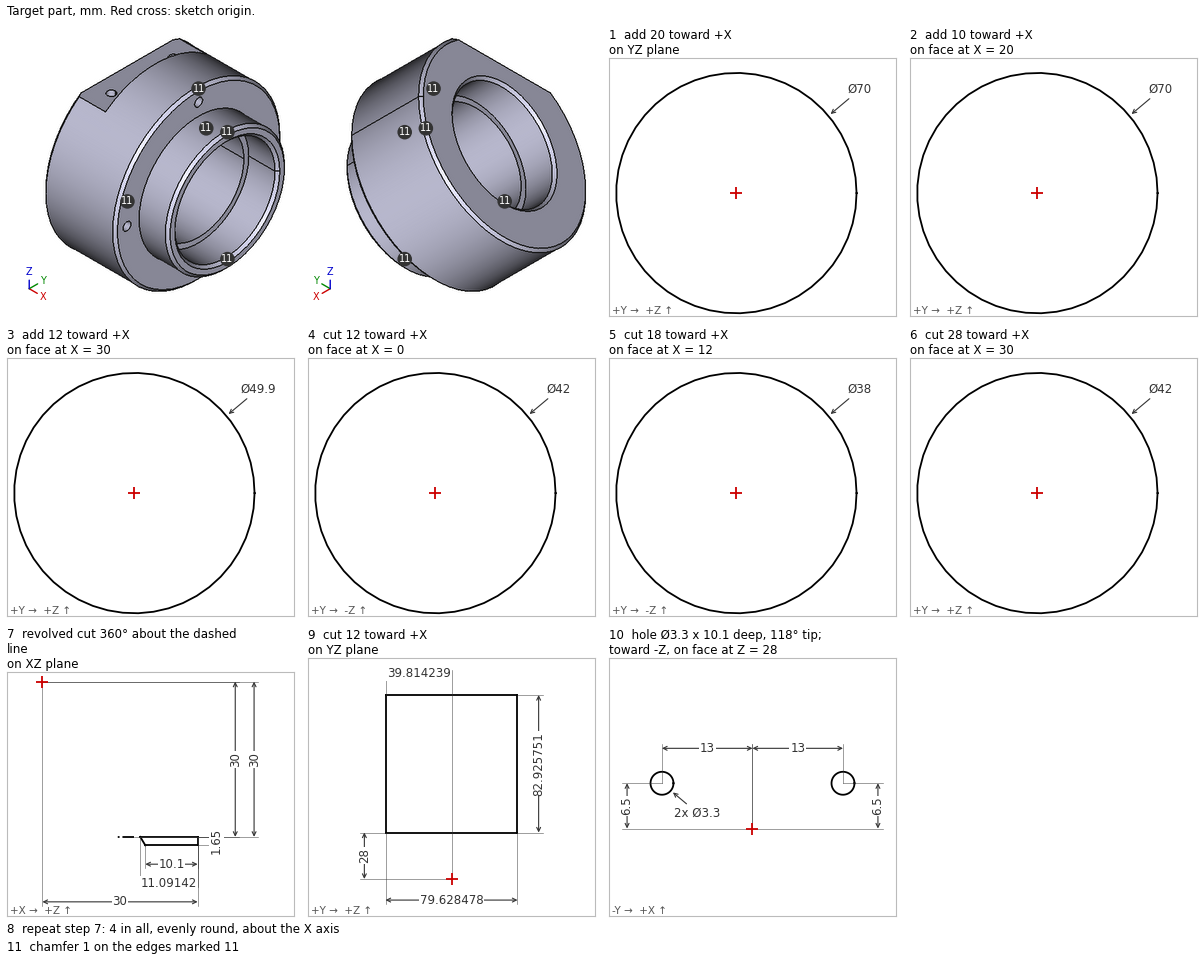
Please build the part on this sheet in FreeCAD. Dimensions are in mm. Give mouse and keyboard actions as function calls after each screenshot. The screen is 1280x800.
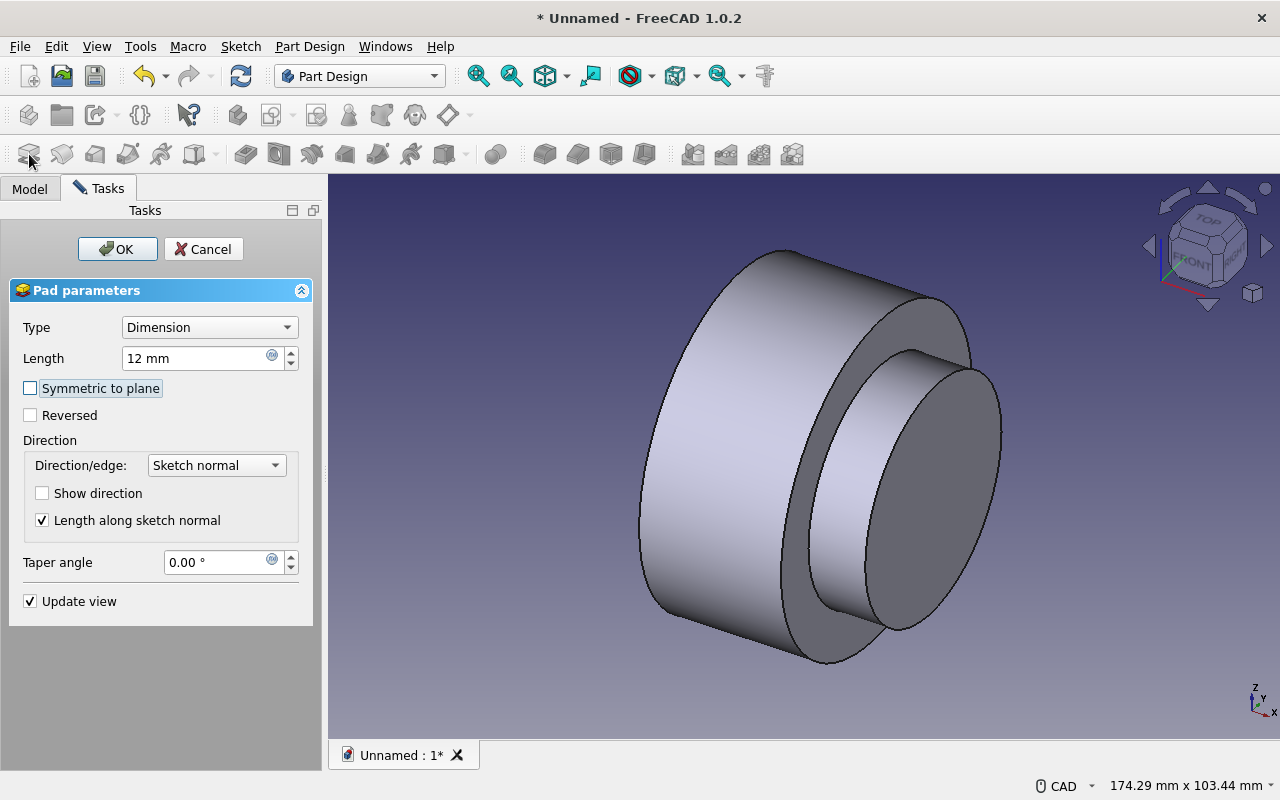
click(118, 249)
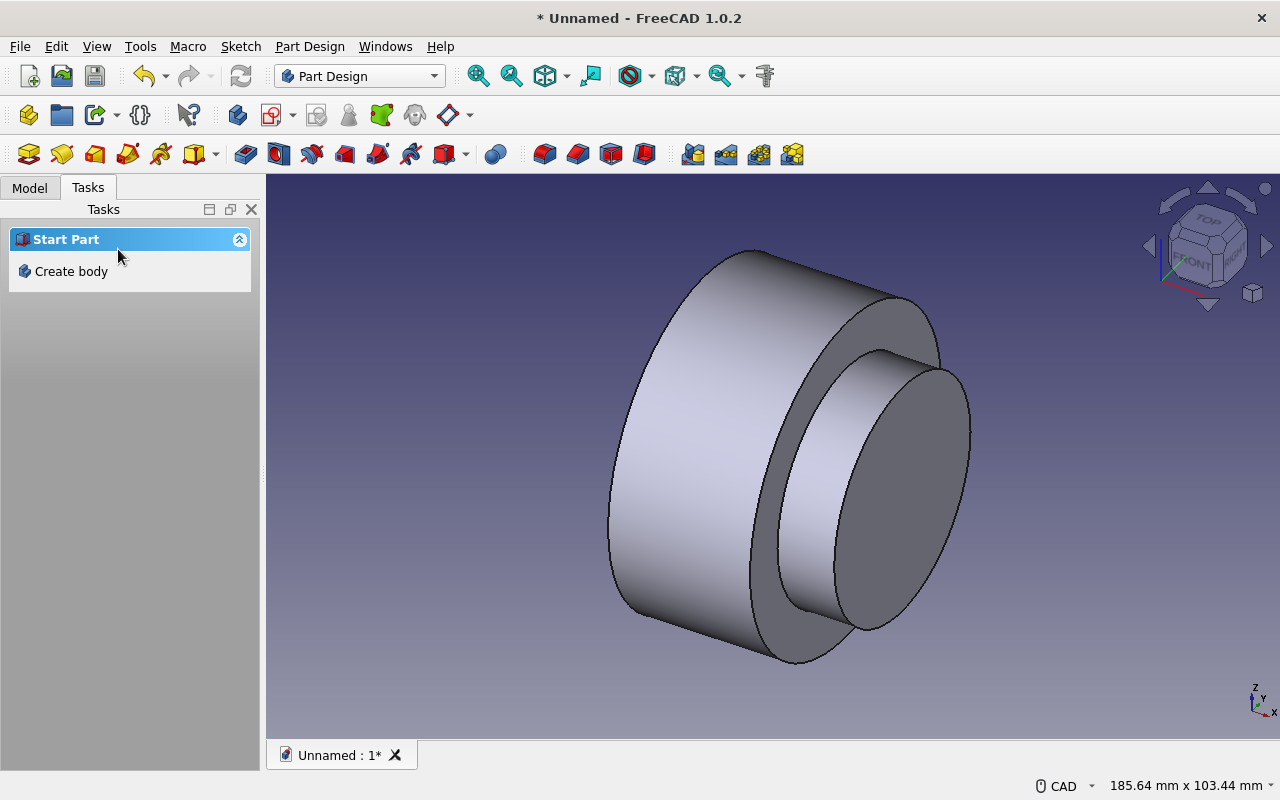
click(479, 76)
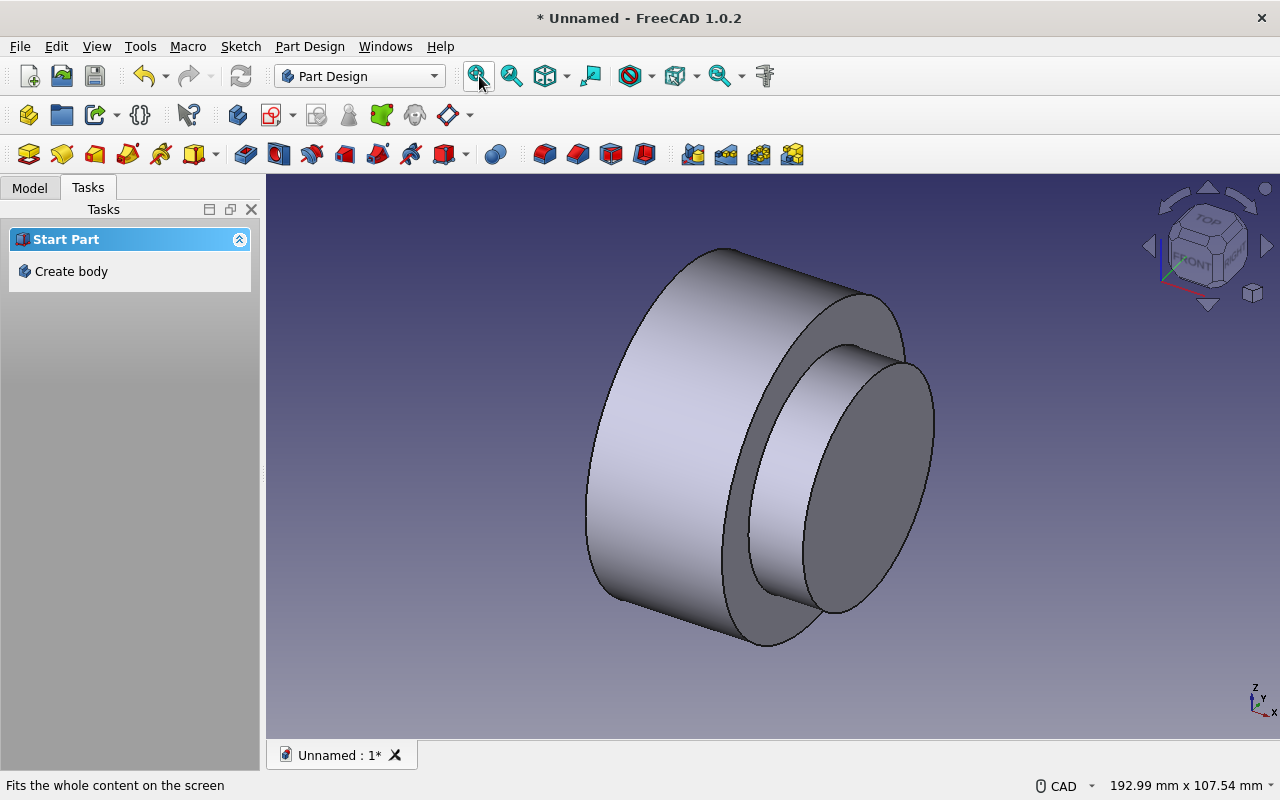
key(6)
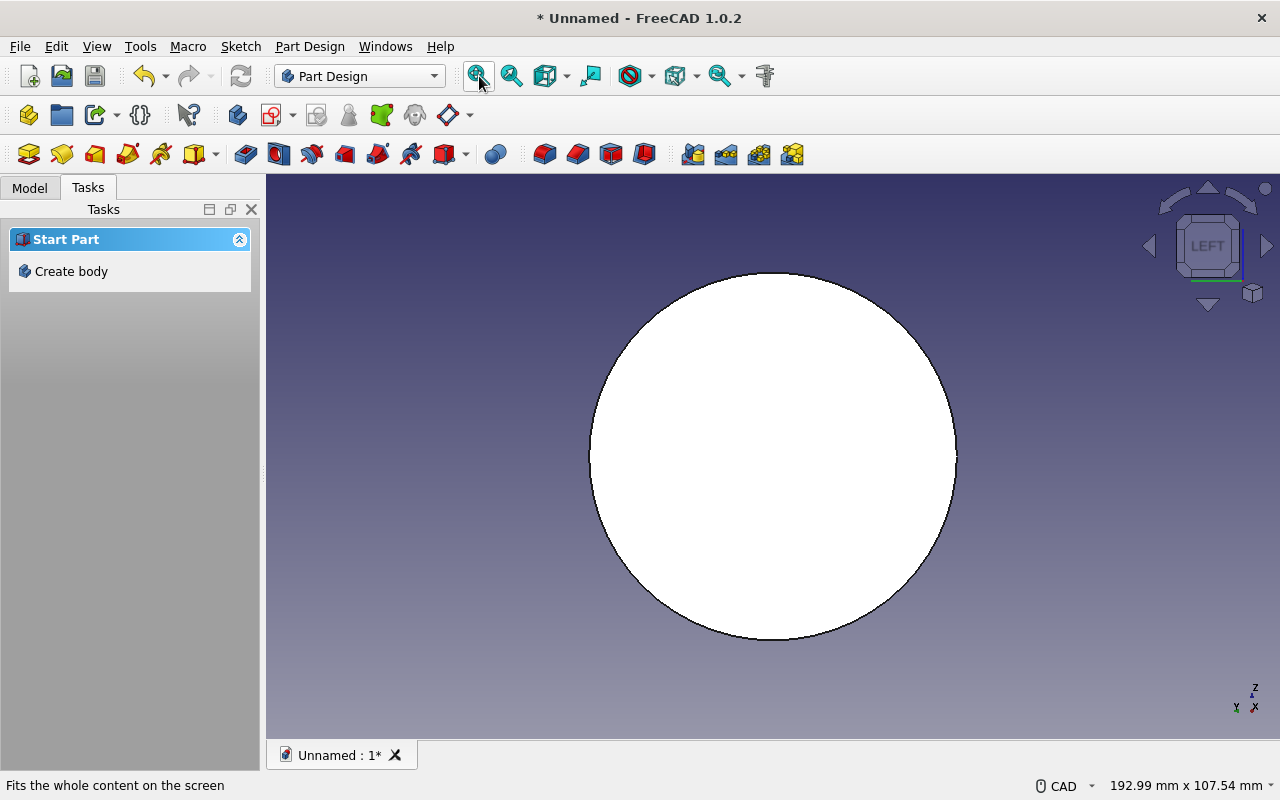
click(773, 455)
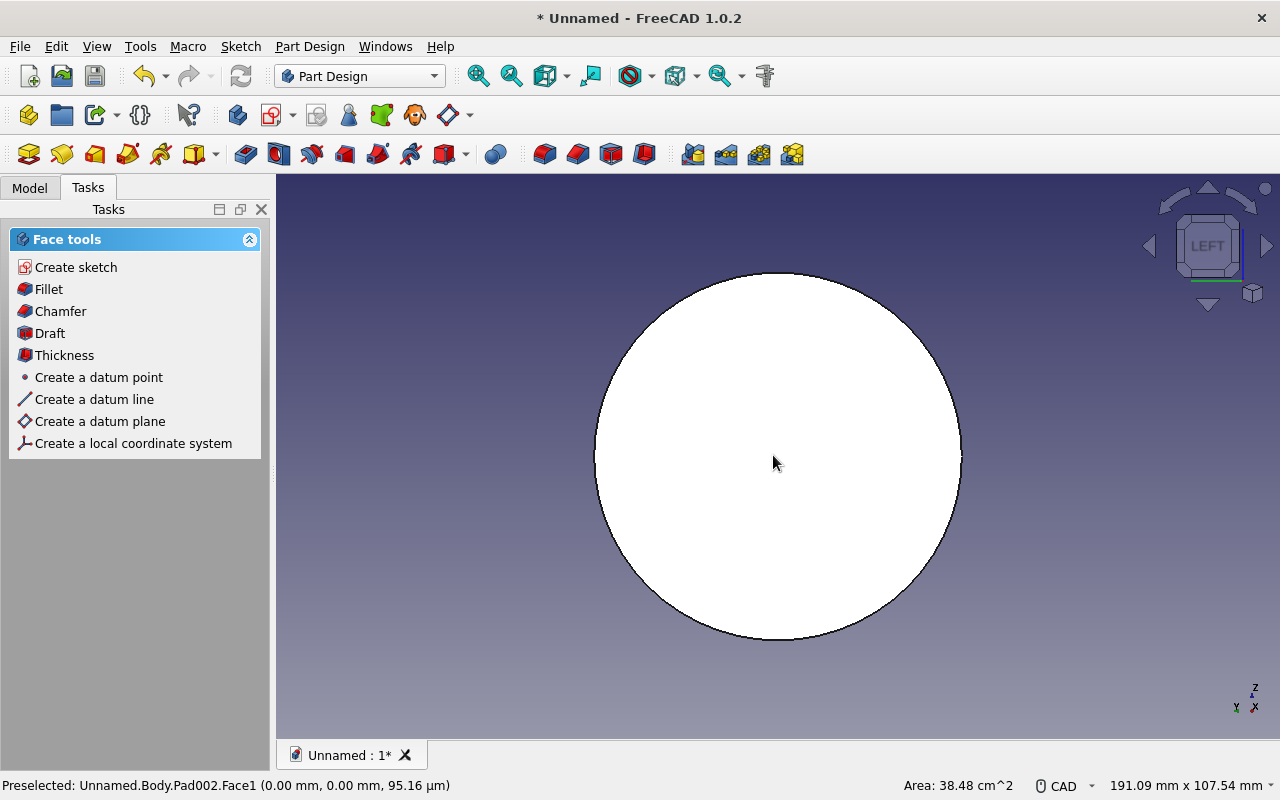
click(270, 116)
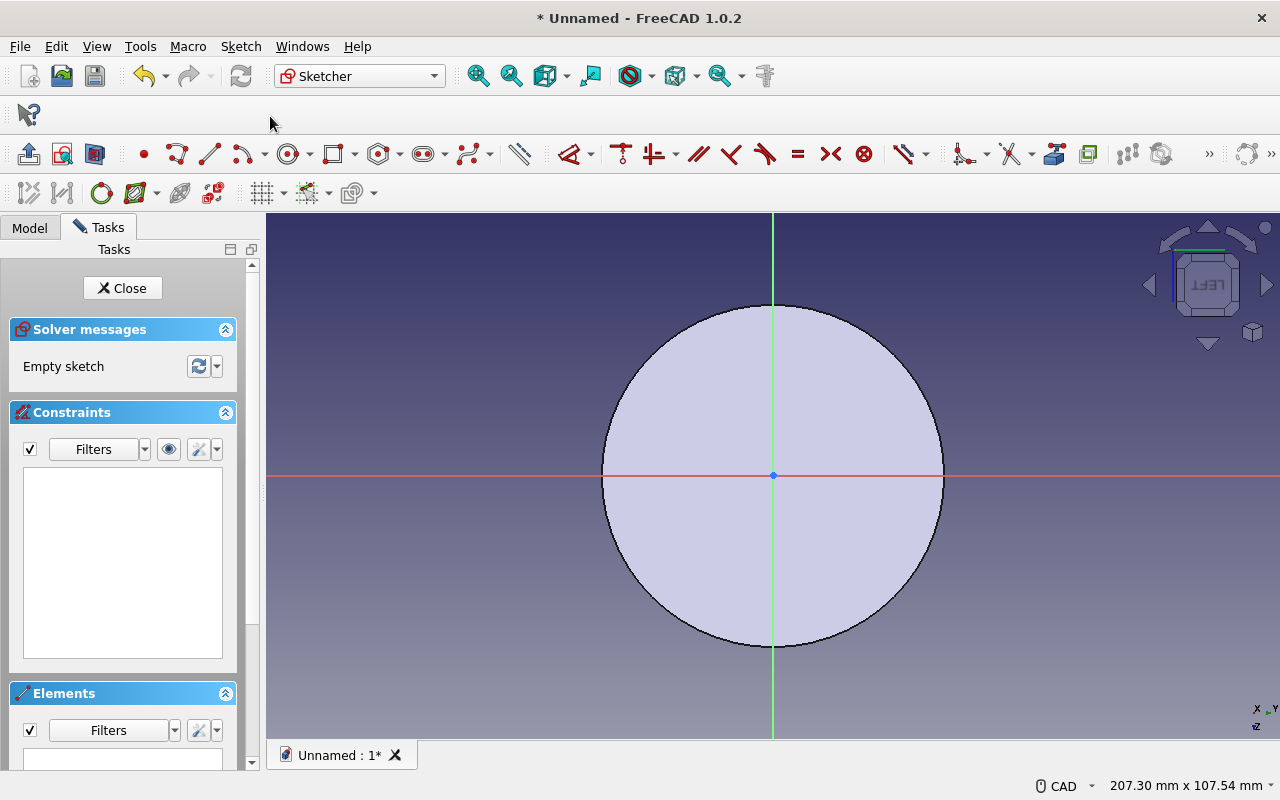
scroll(912, 476, up, 2)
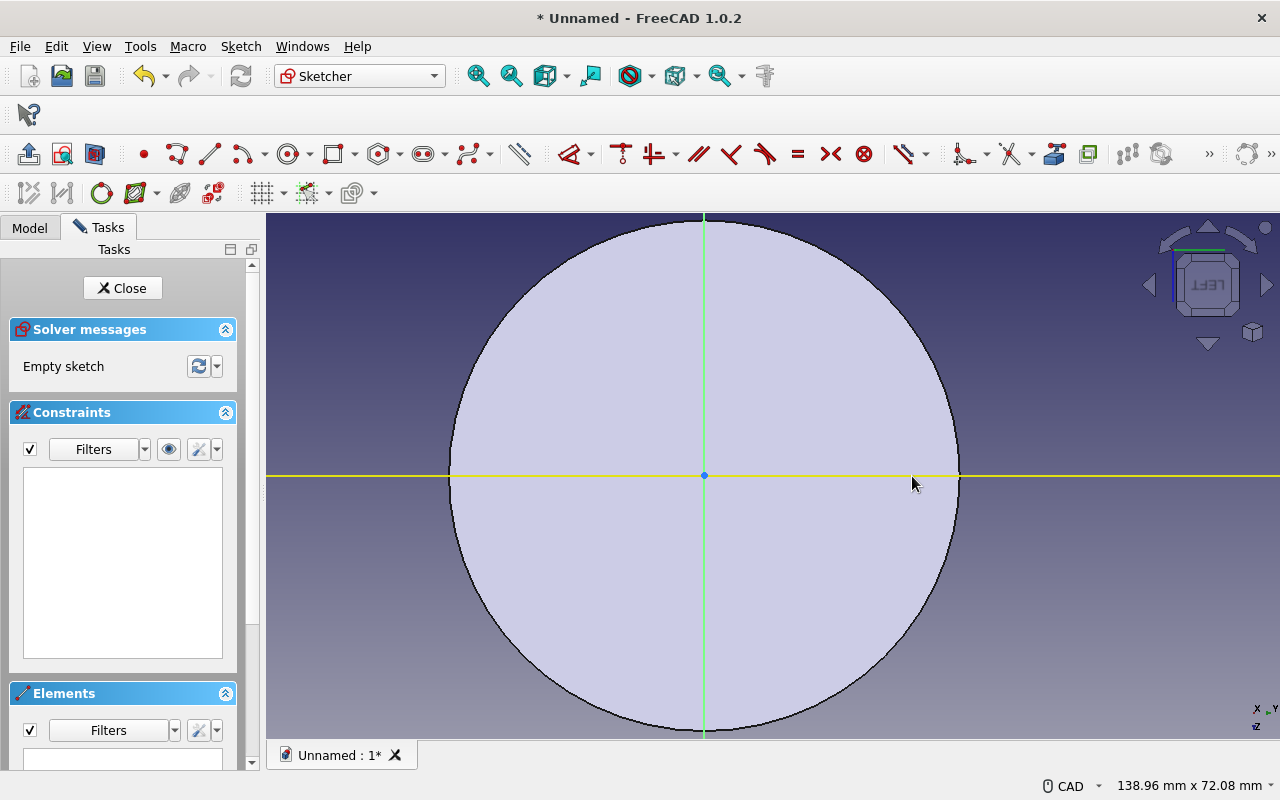
key(g)
key(c)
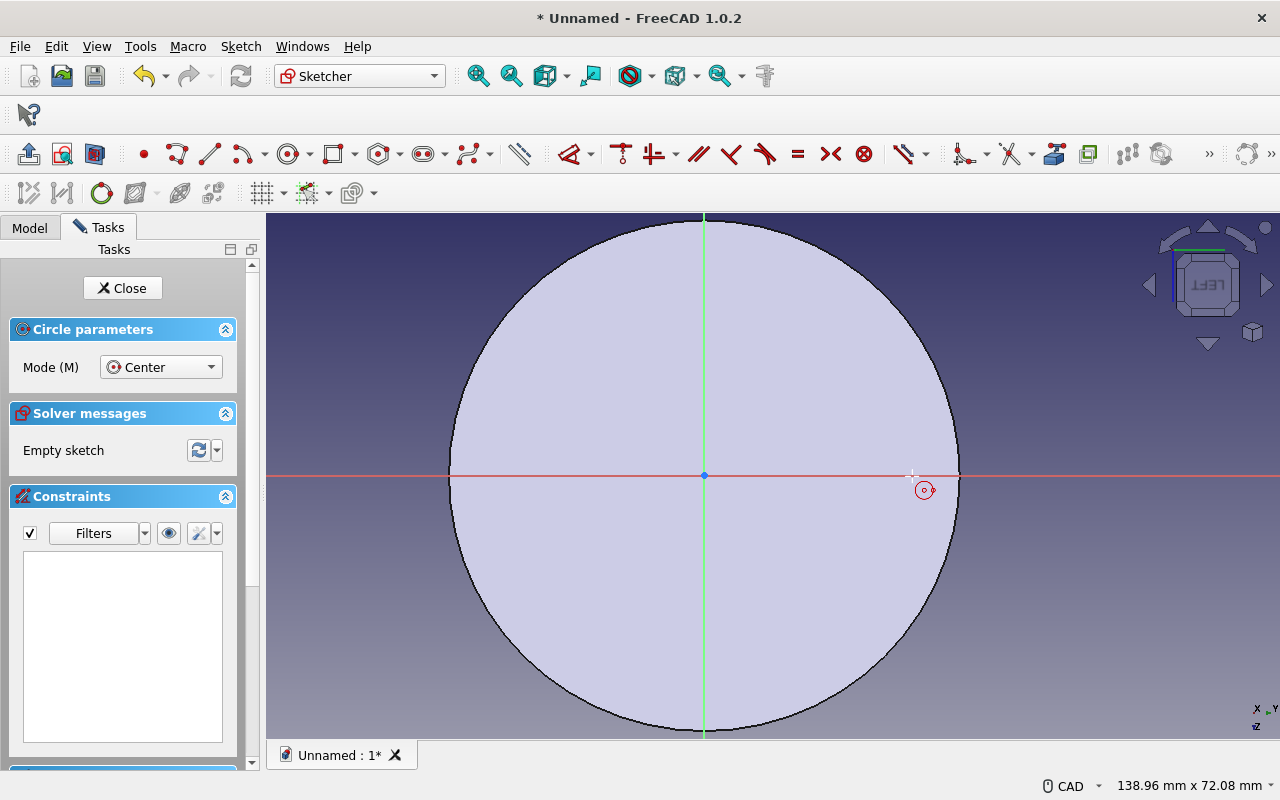
click(704, 476)
move(813, 367)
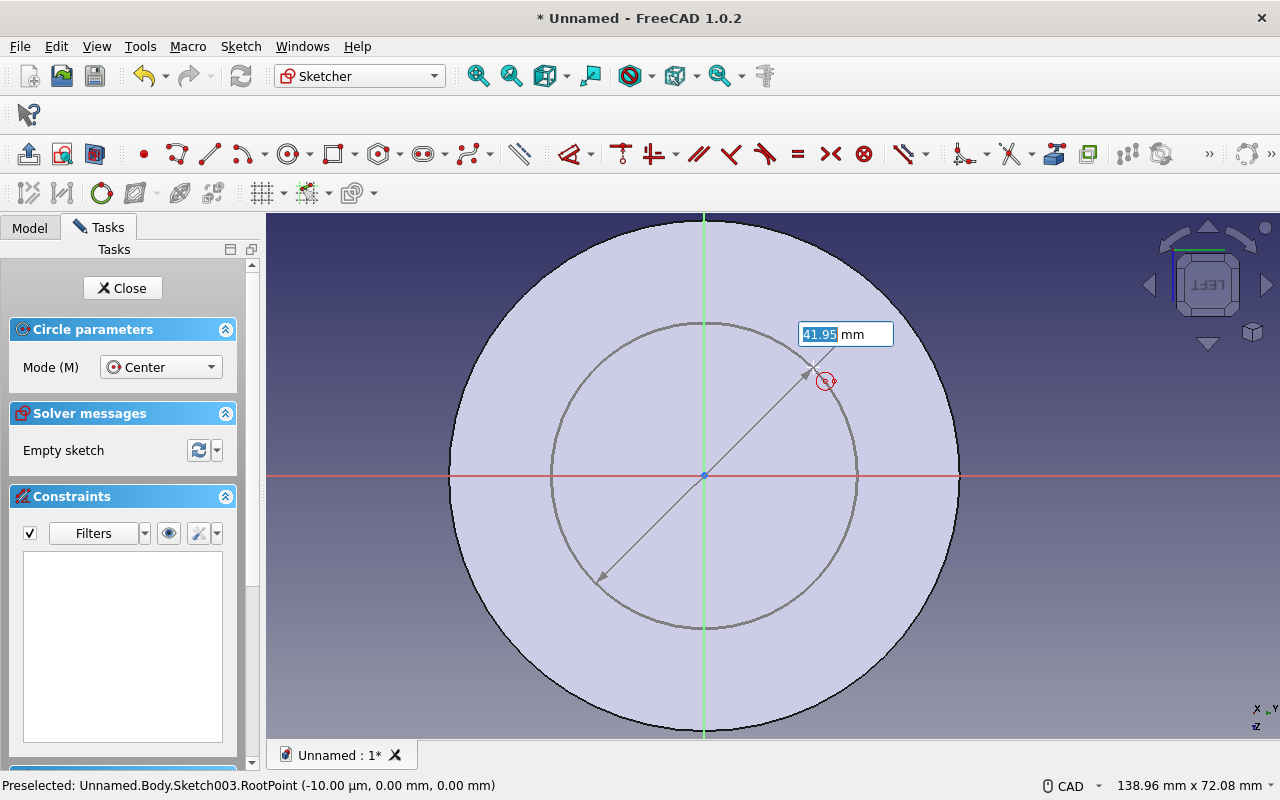
text(42)
key(Return)
key(Escape)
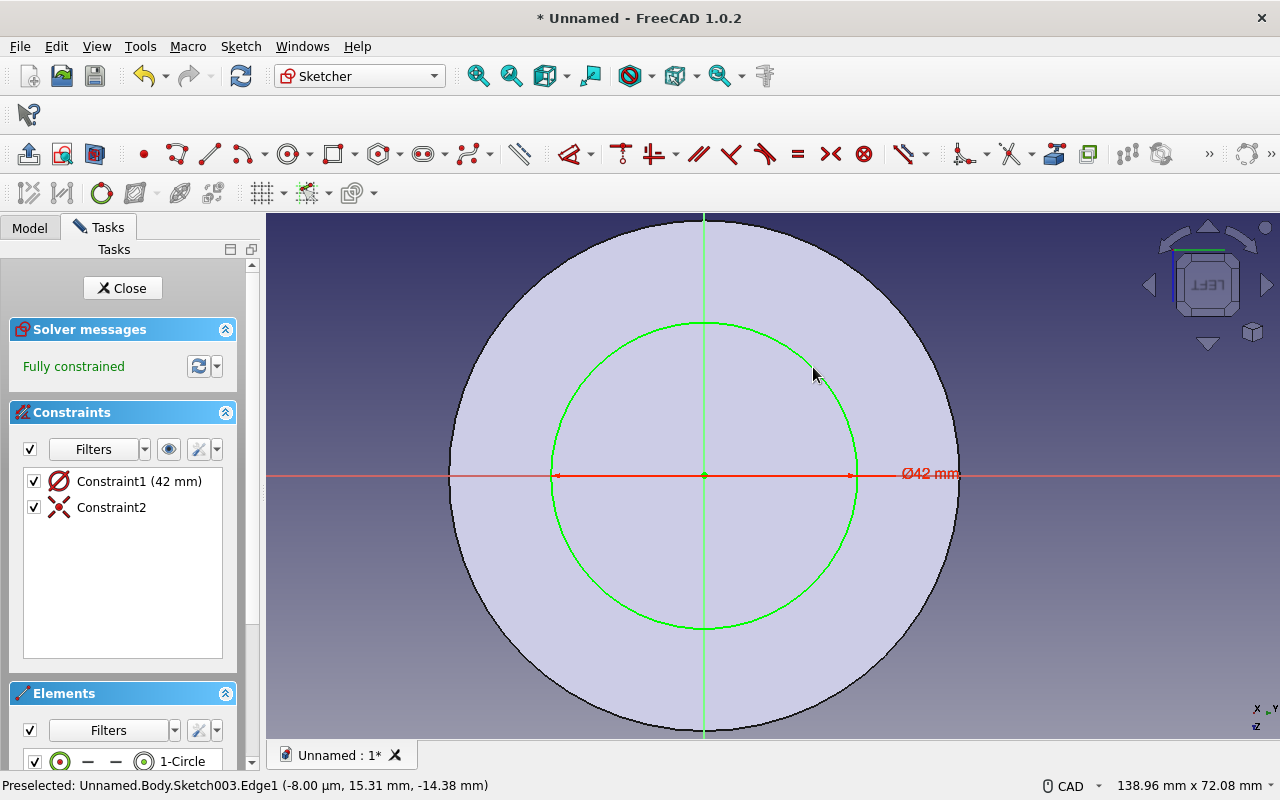
click(123, 288)